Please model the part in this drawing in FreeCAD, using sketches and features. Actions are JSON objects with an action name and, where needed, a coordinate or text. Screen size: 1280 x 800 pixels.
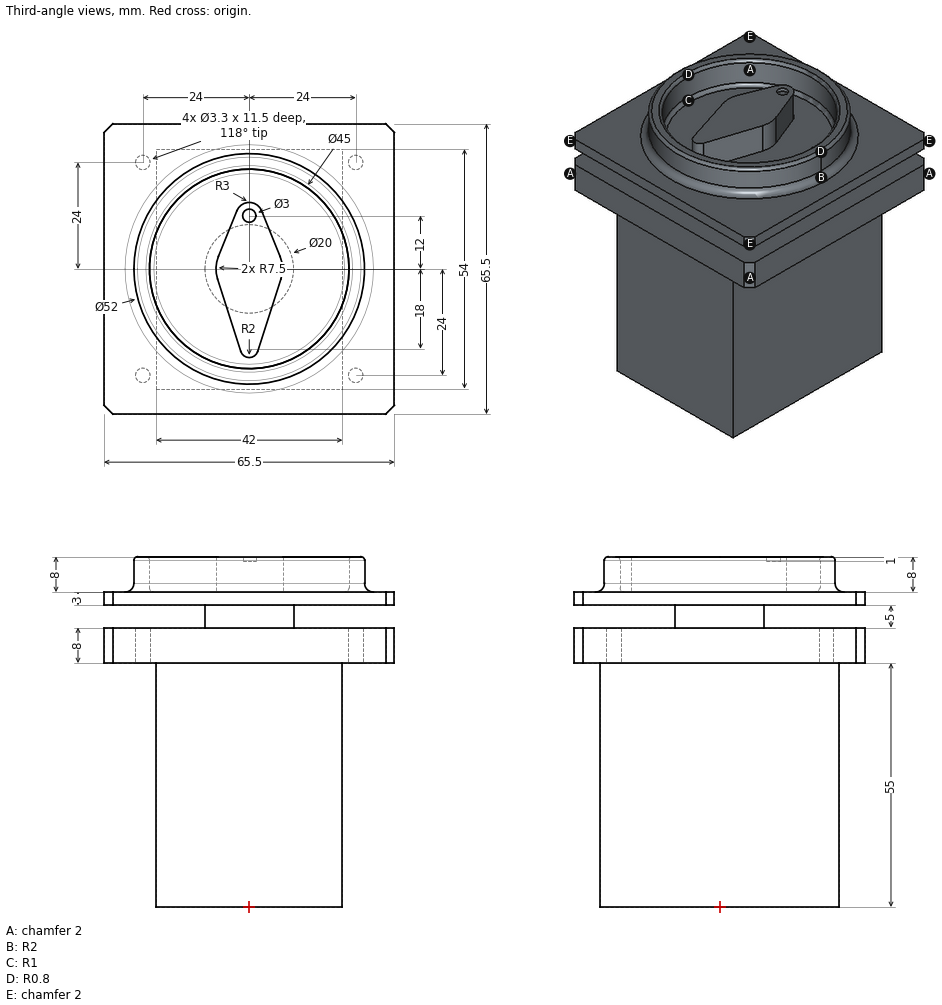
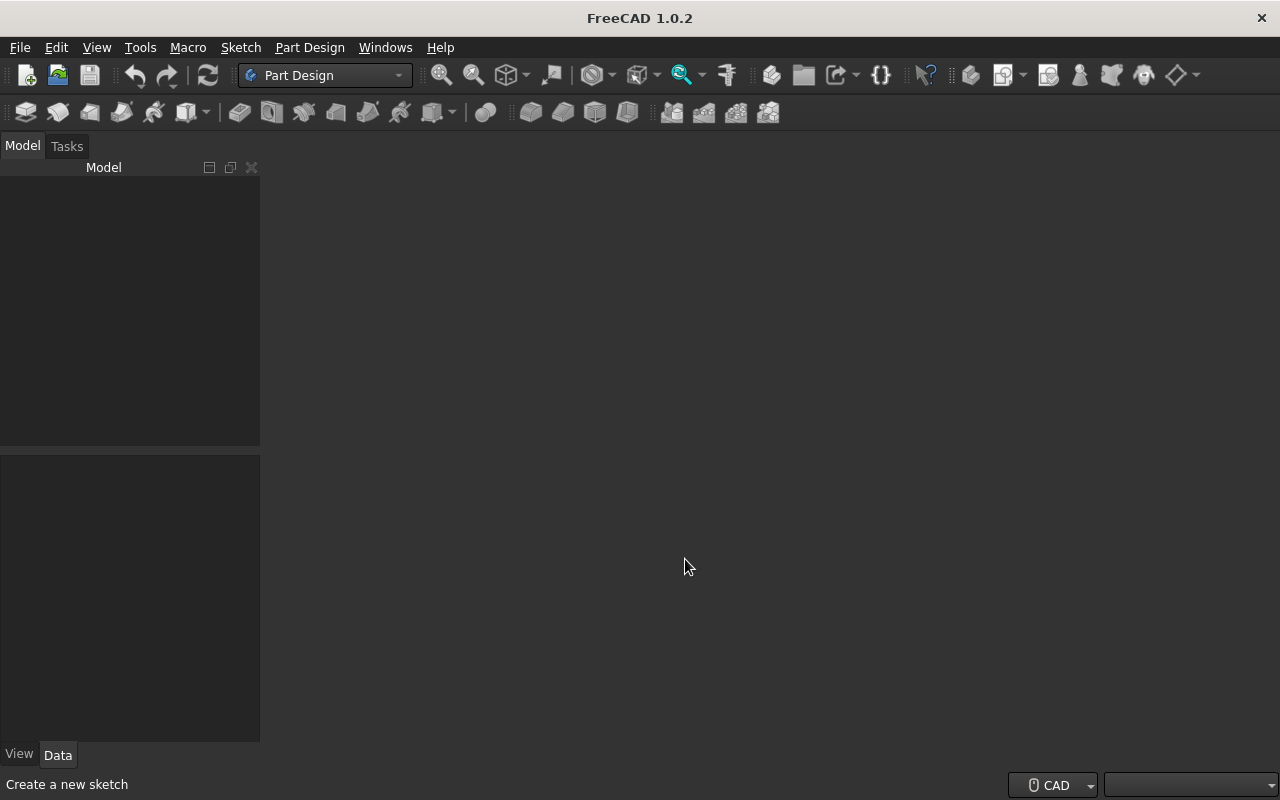
{"action": "left_click", "coordinate": [26, 76]}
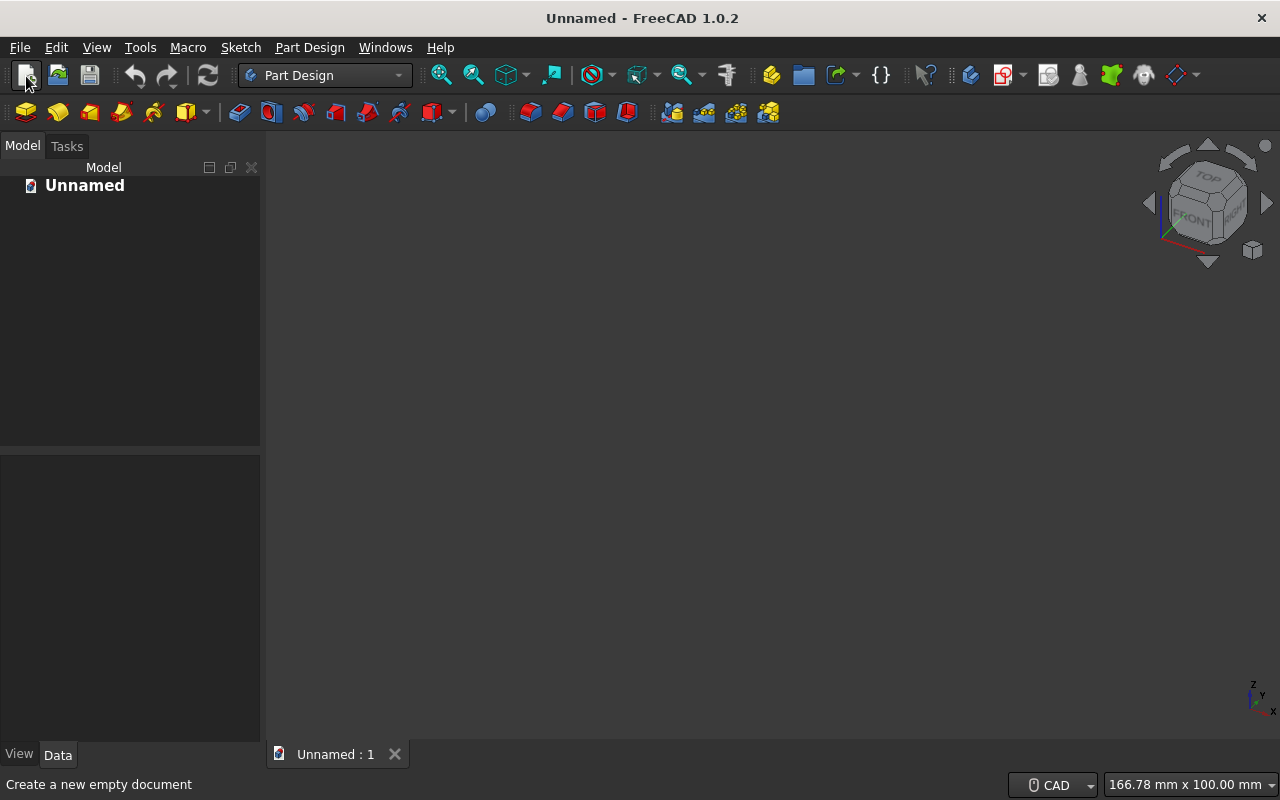
{"action": "left_click", "coordinate": [1004, 76]}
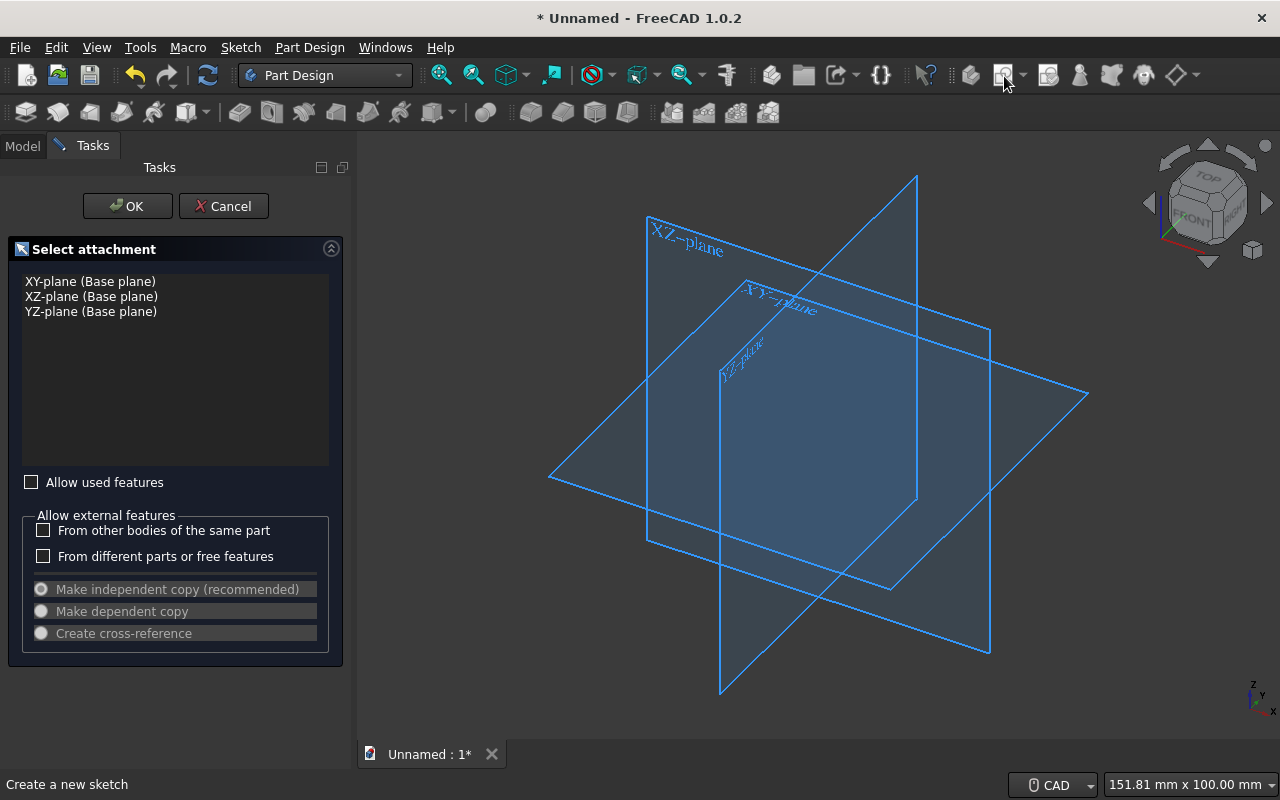
{"action": "left_click", "coordinate": [82, 282]}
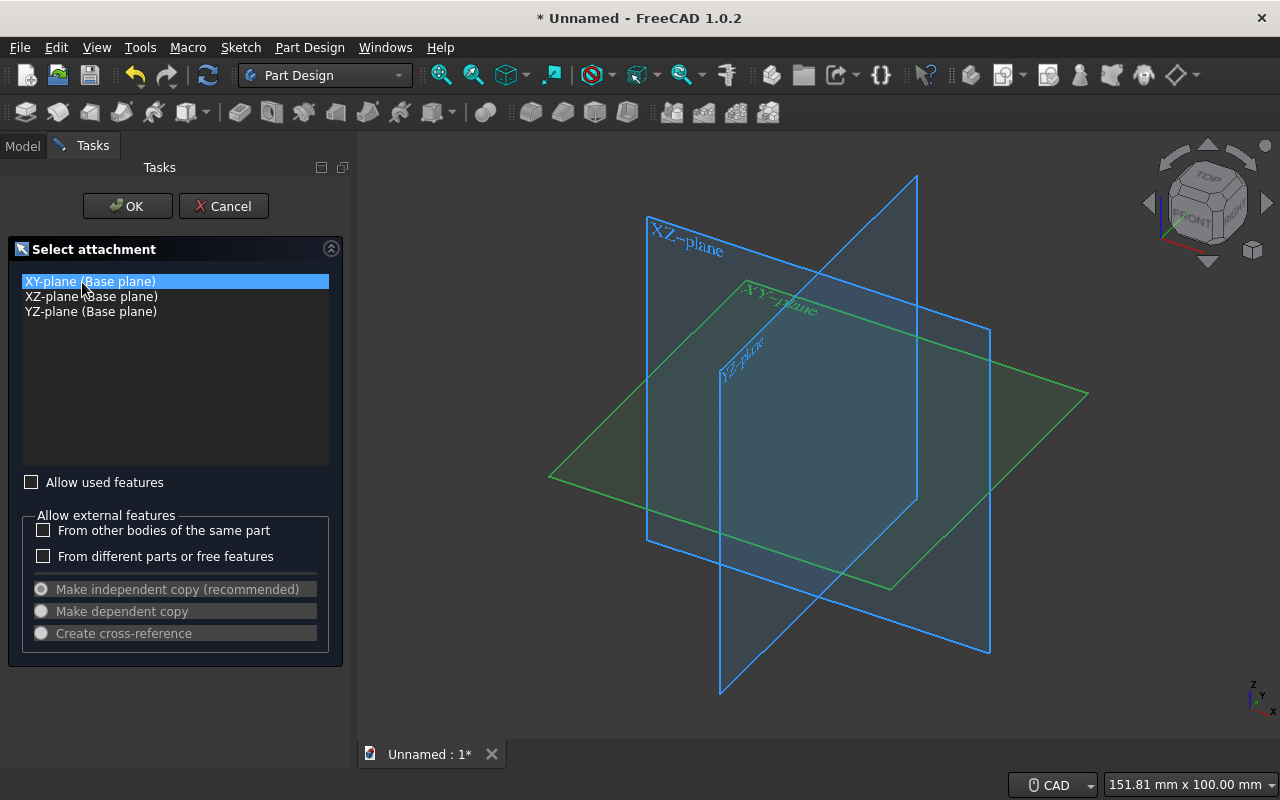
{"action": "left_click", "coordinate": [128, 206]}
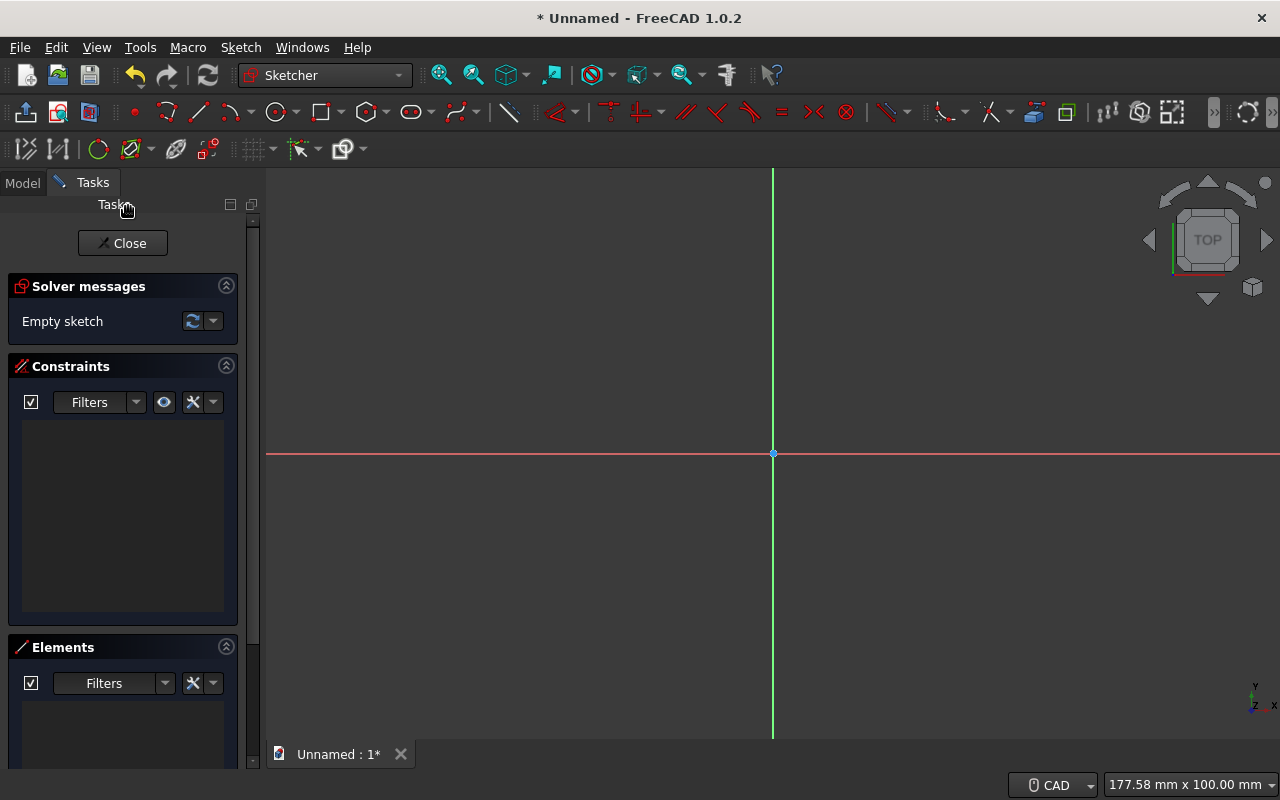
{"action": "key", "text": "g v"}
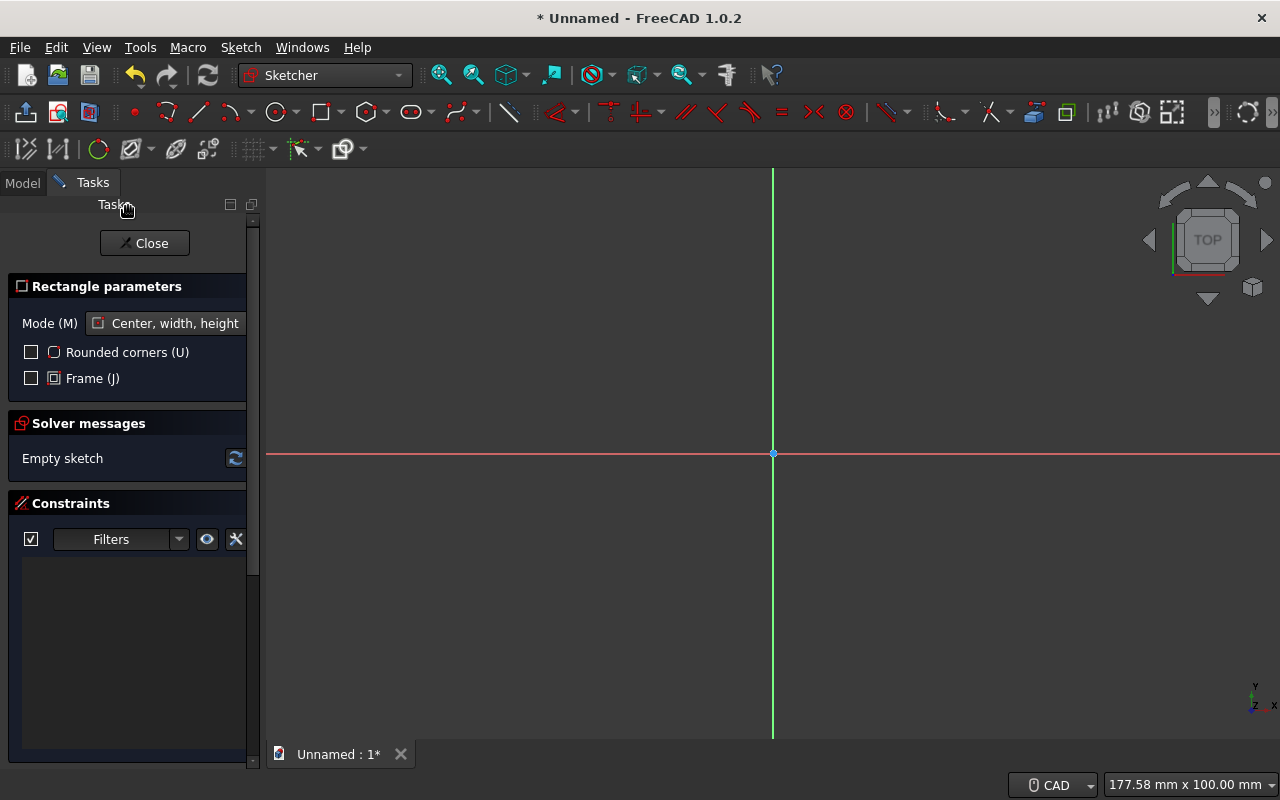
{"action": "left_click", "coordinate": [773, 454]}
{"action": "mouse_move", "coordinate": [893, 299]}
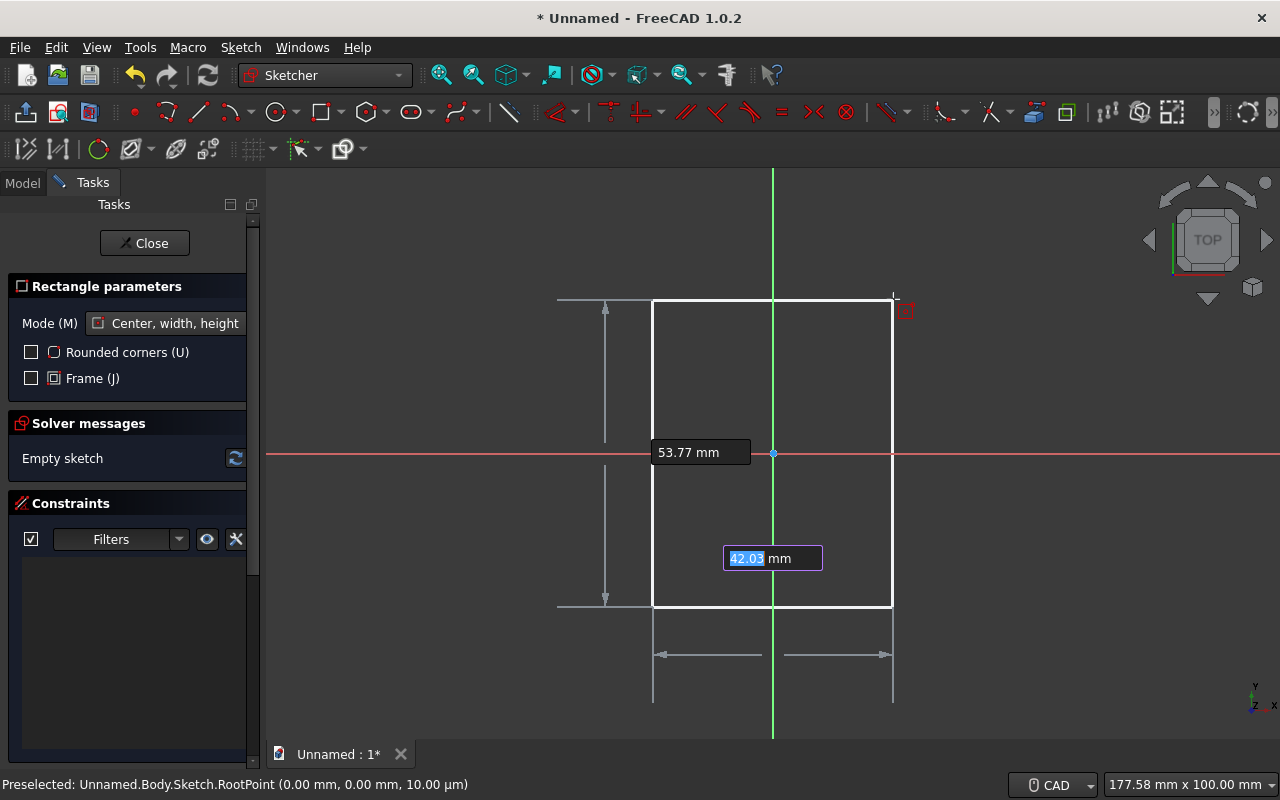
{"action": "type", "text": "42"}
{"action": "key", "text": "Tab"}
{"action": "type", "text": "54"}
{"action": "key", "text": "Return"}
{"action": "key", "text": "Escape"}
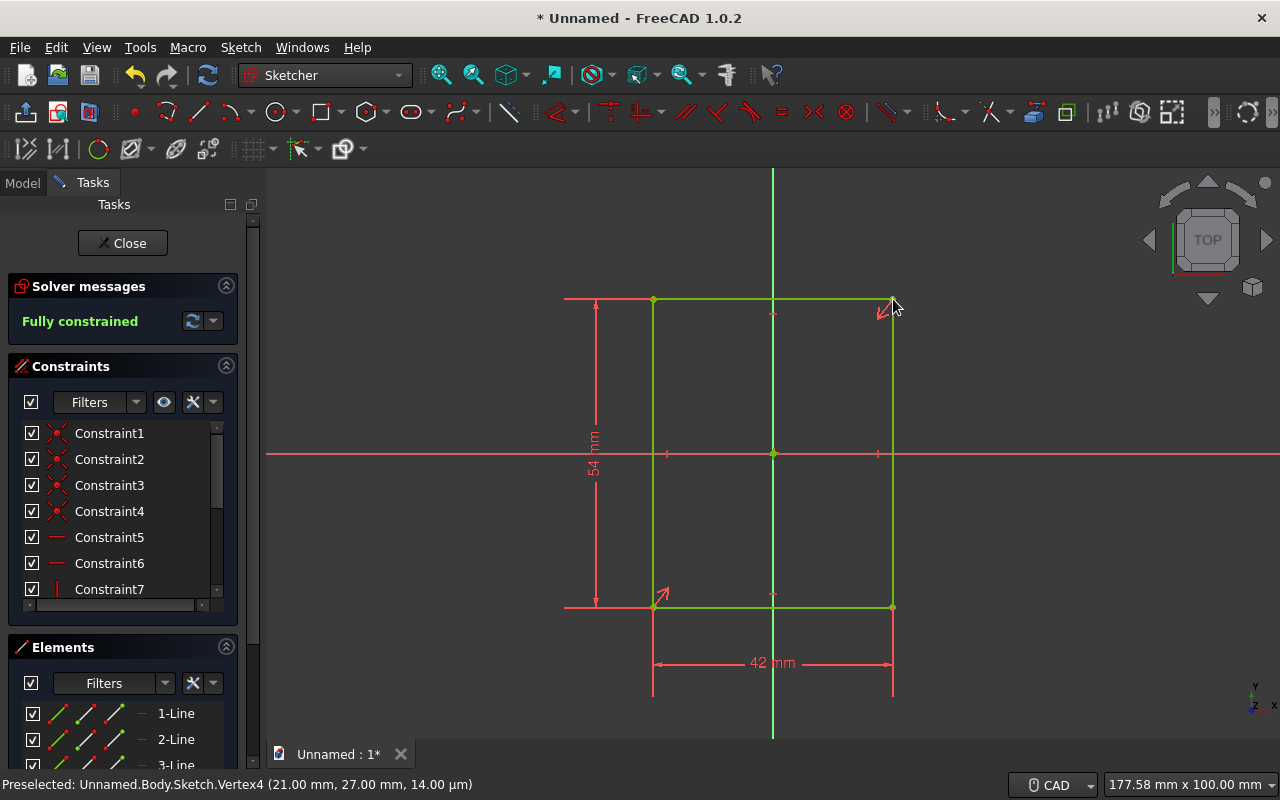
{"action": "left_click", "coordinate": [123, 243]}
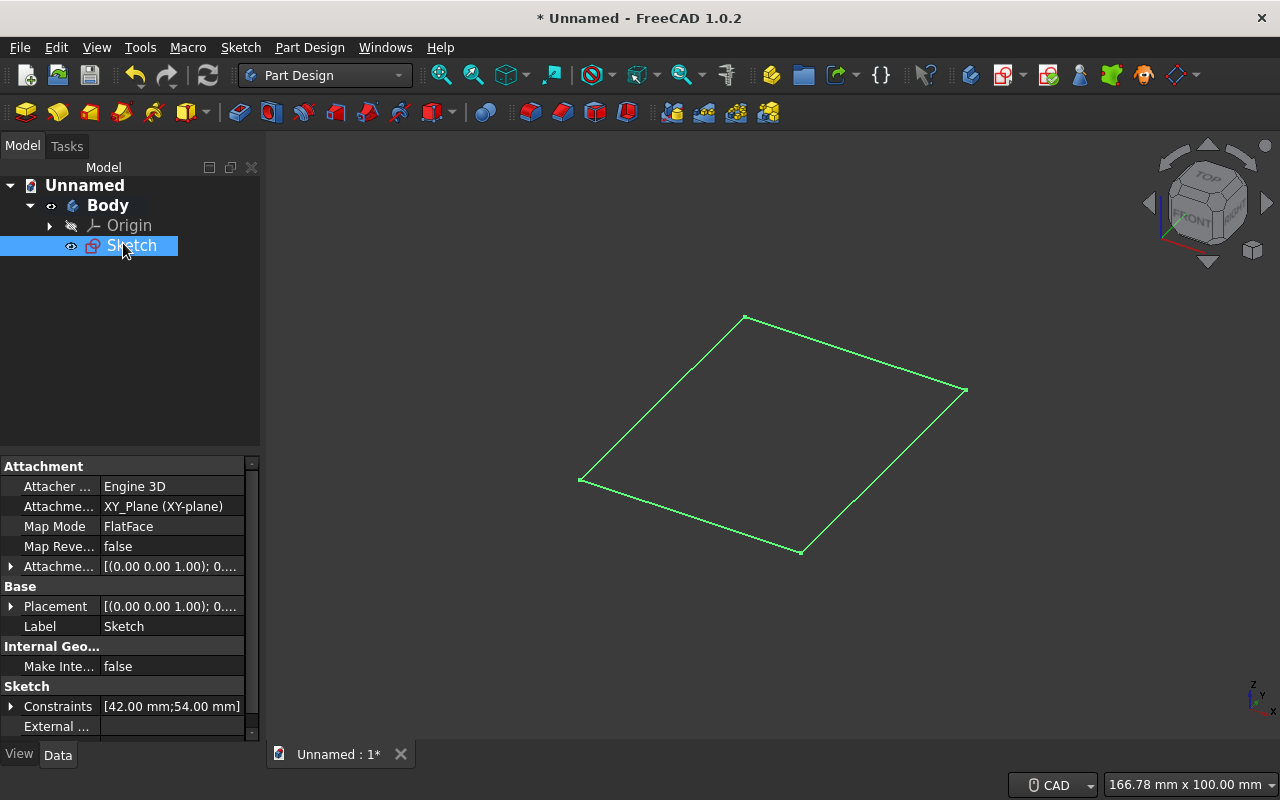
{"action": "left_click", "coordinate": [26, 112]}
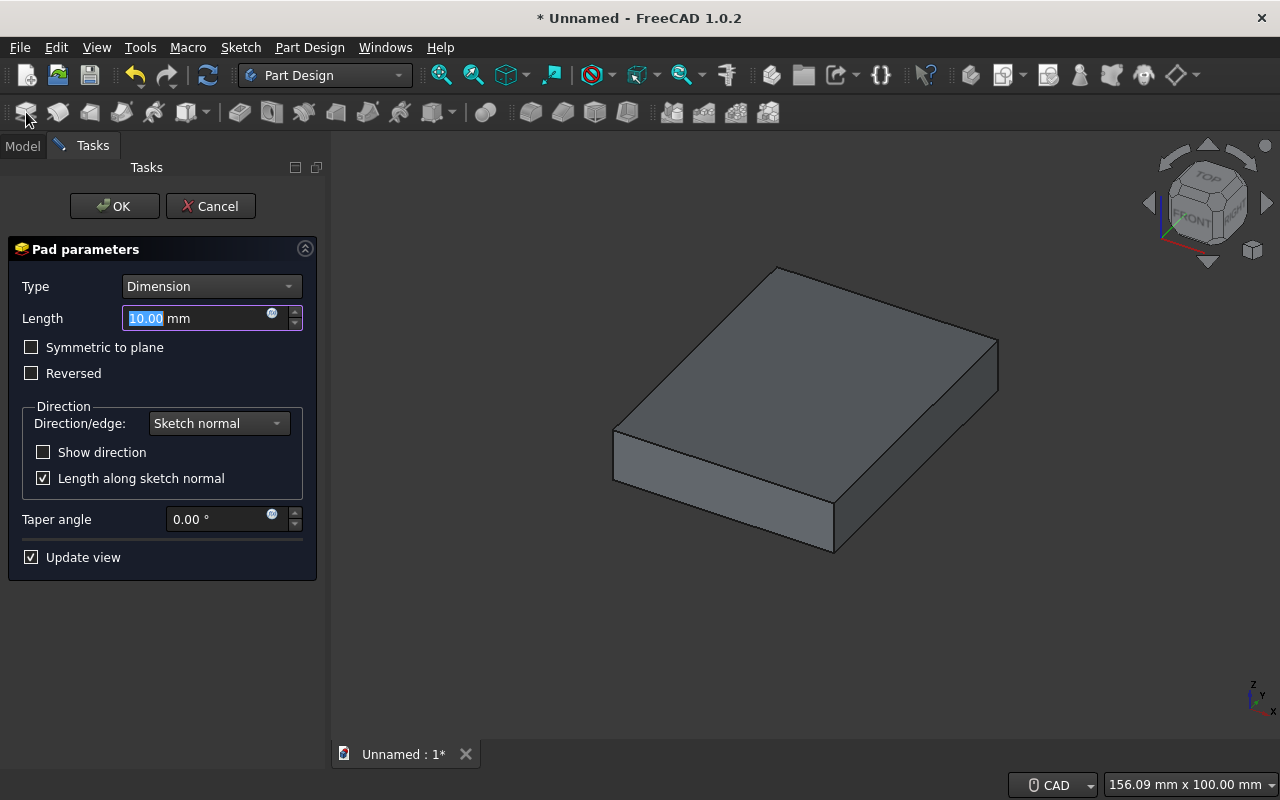
{"action": "type", "text": "55"}
{"action": "key", "text": "Tab"}